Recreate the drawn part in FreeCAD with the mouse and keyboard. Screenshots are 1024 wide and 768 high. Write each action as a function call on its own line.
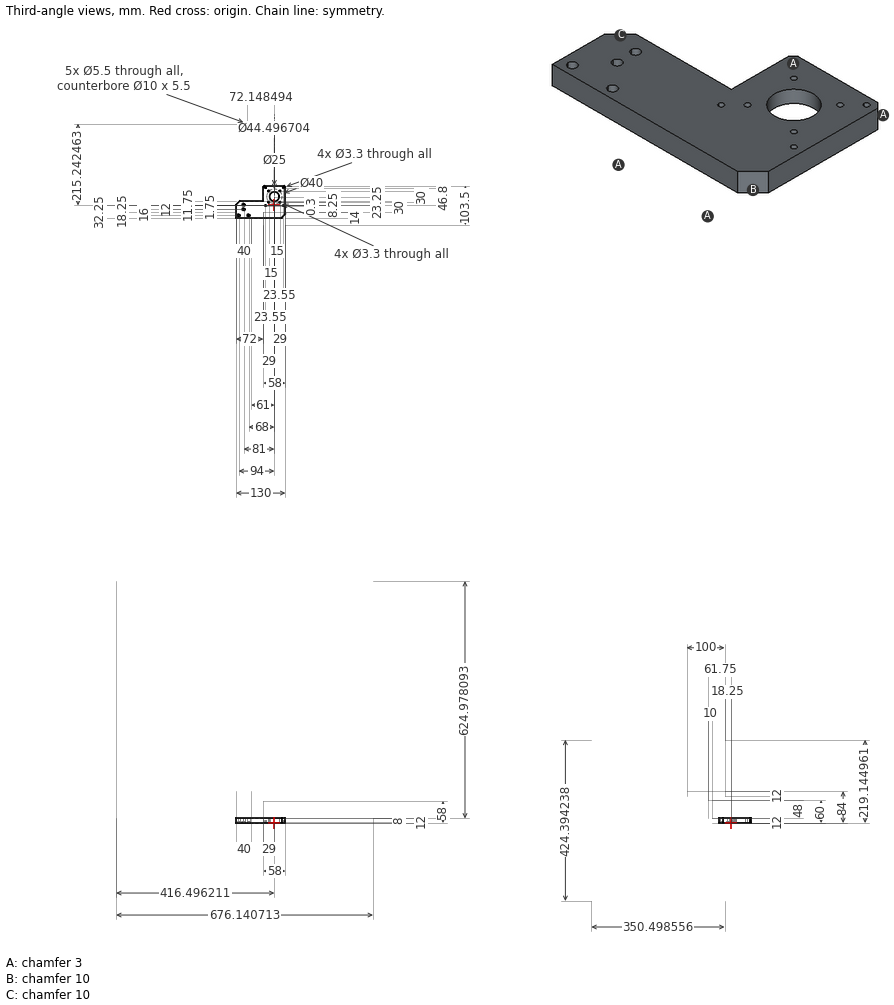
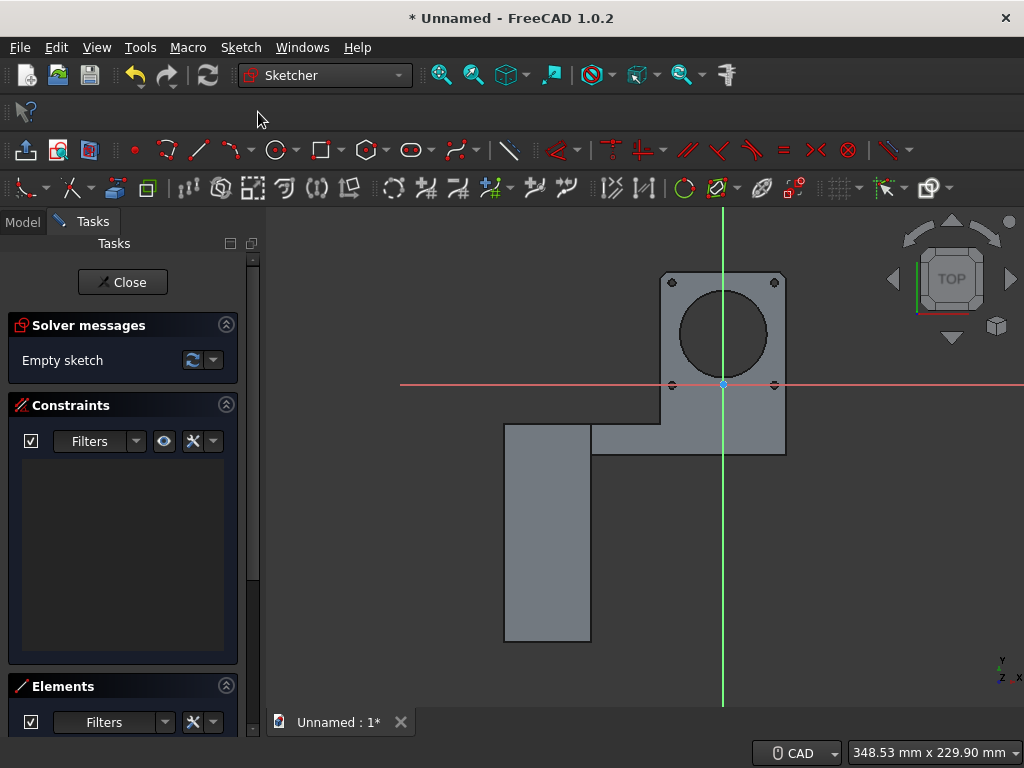
click(90, 150)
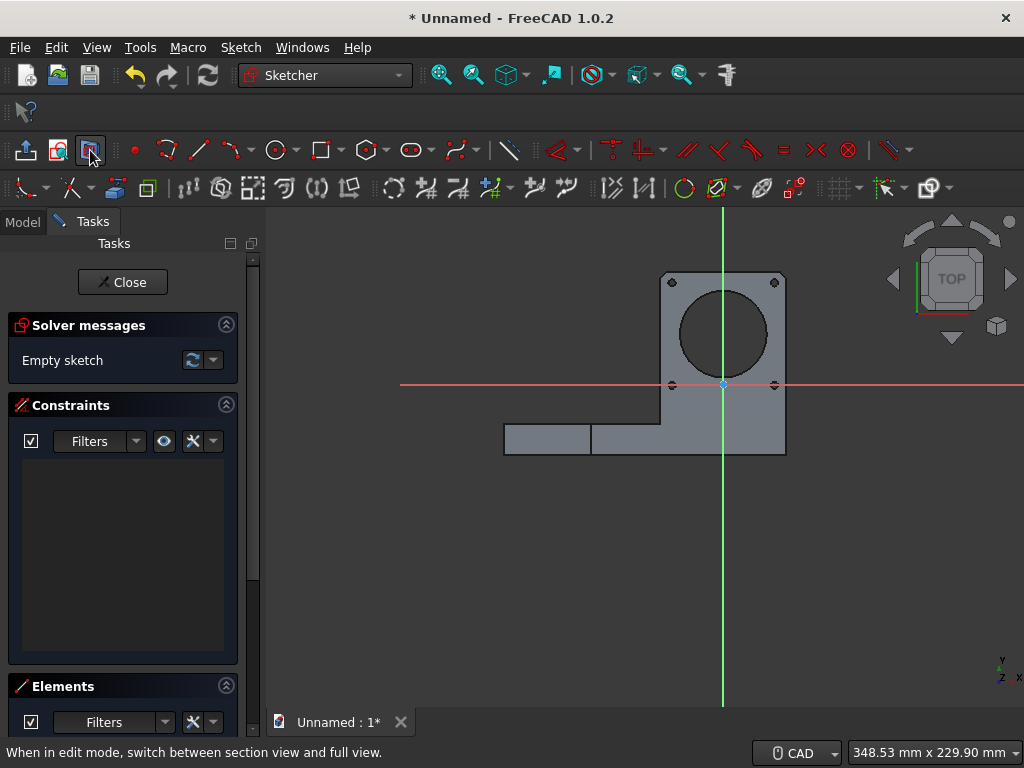
scroll(658, 312, up, 3)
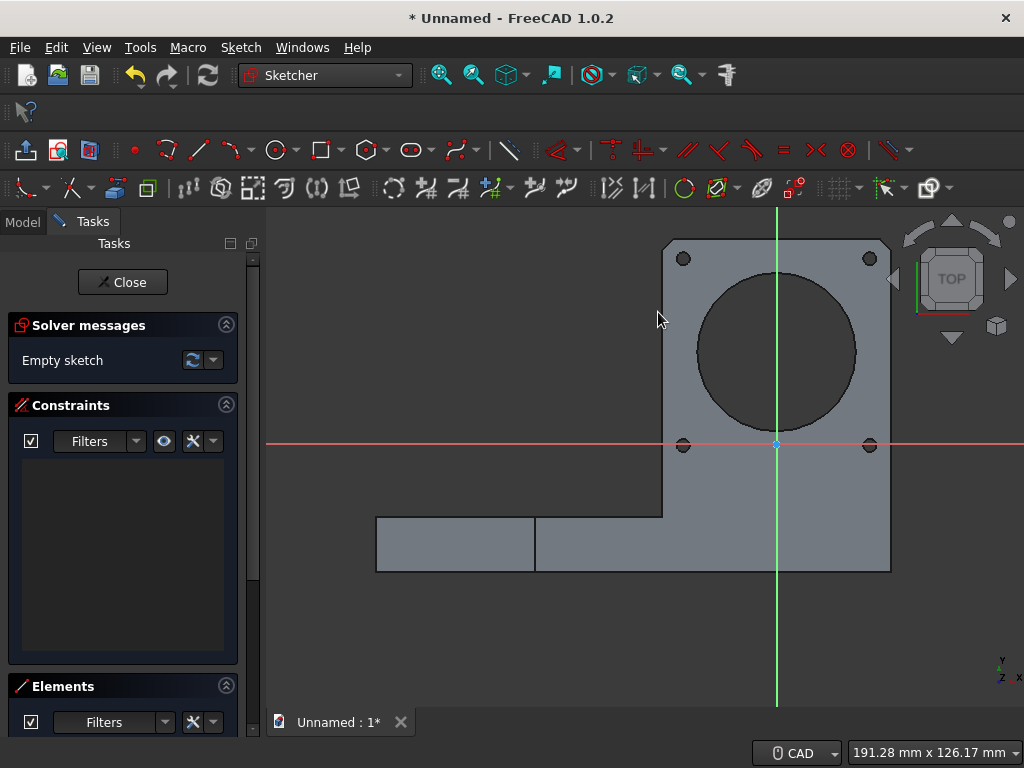
key(g)
key(r)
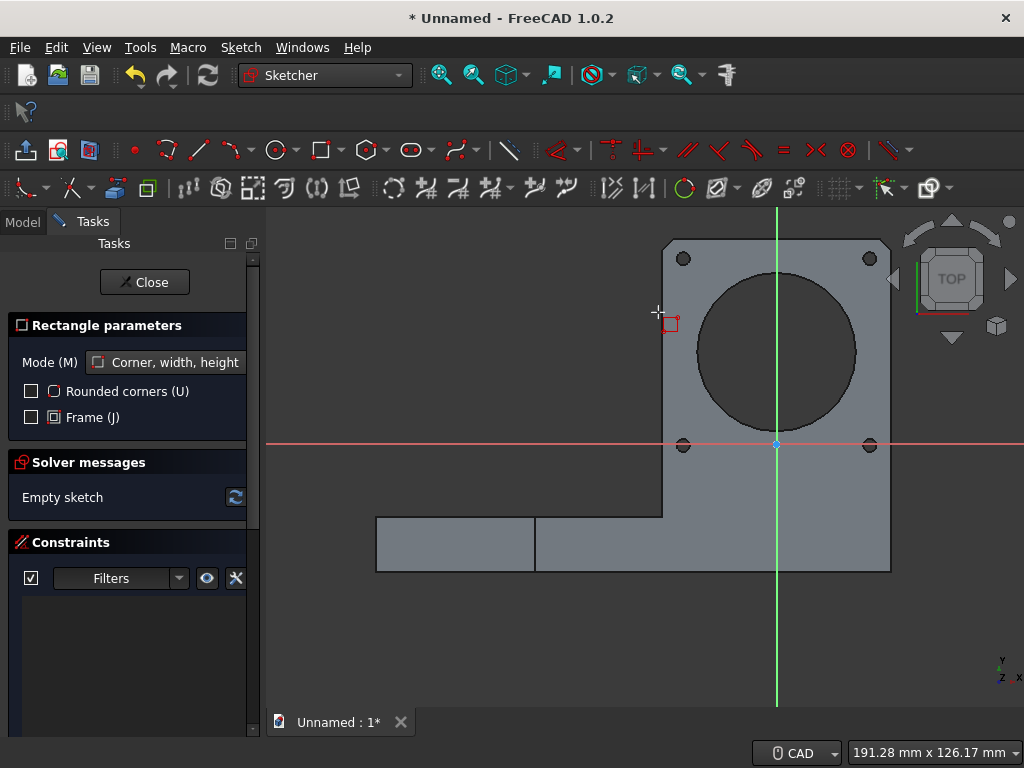
click(376, 398)
move(662, 517)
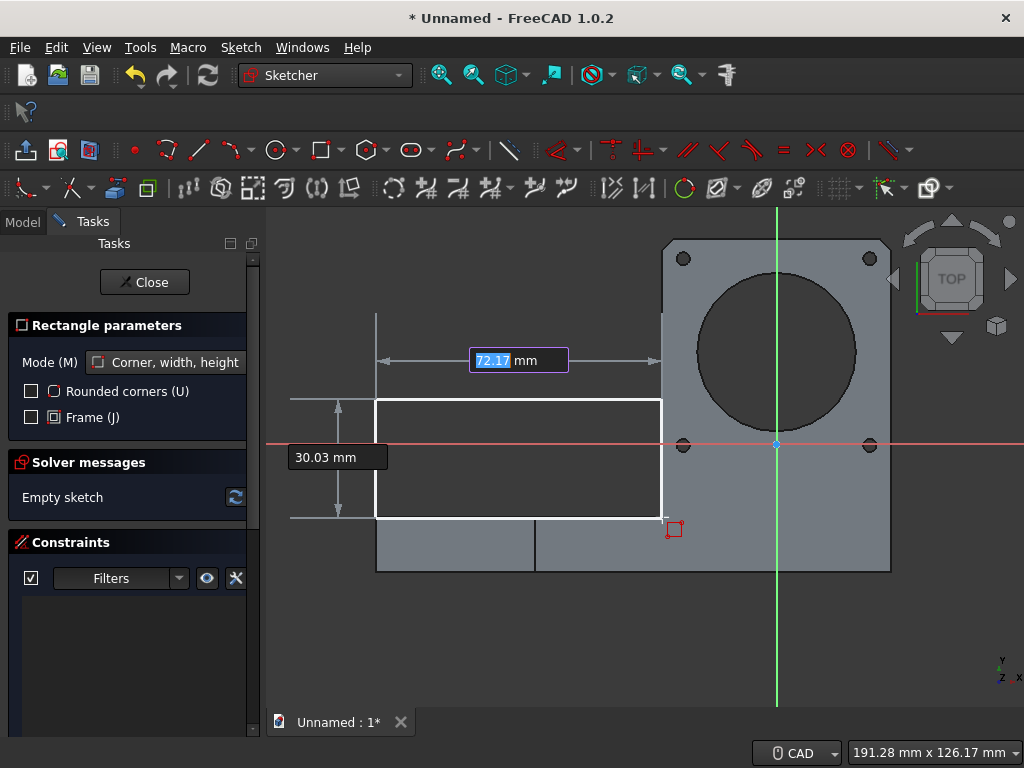
text(72)
key(Tab)
text(30)
key(Return)
key(Escape)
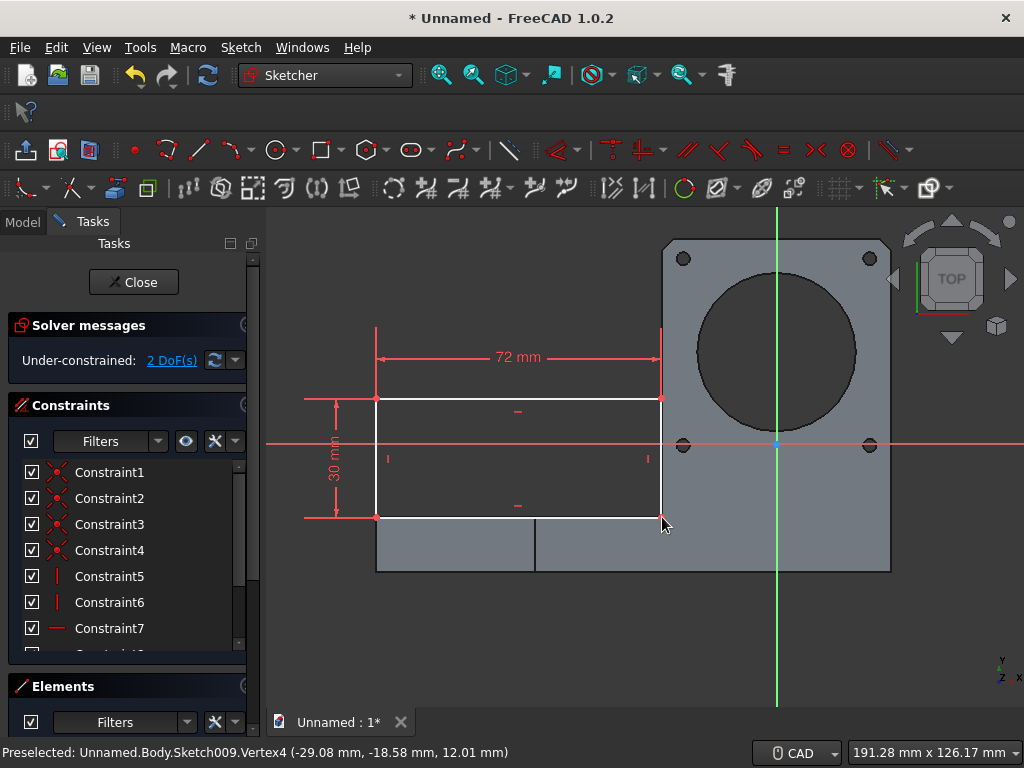
click(556, 150)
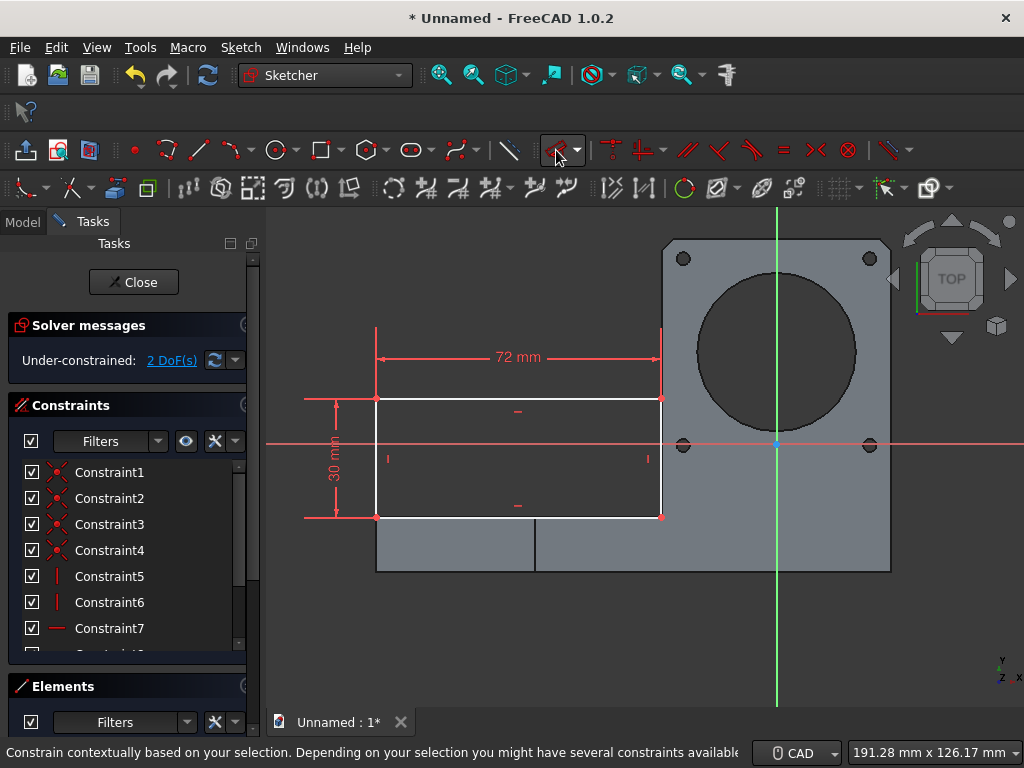
click(661, 518)
click(719, 552)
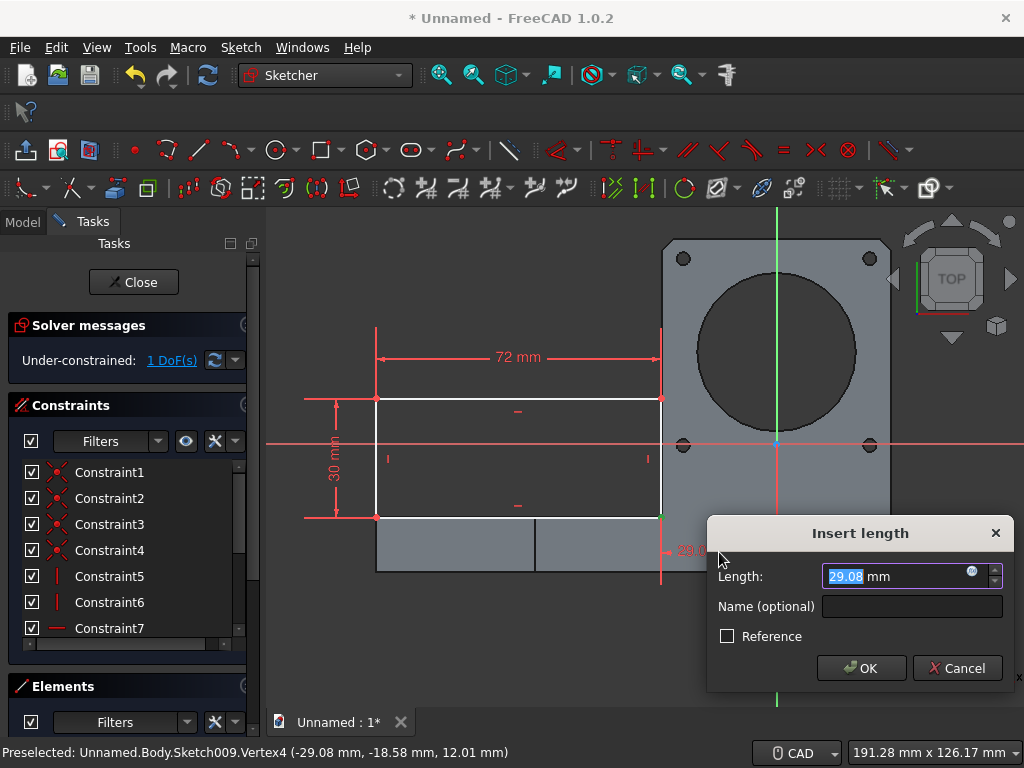
text(29)
key(Return)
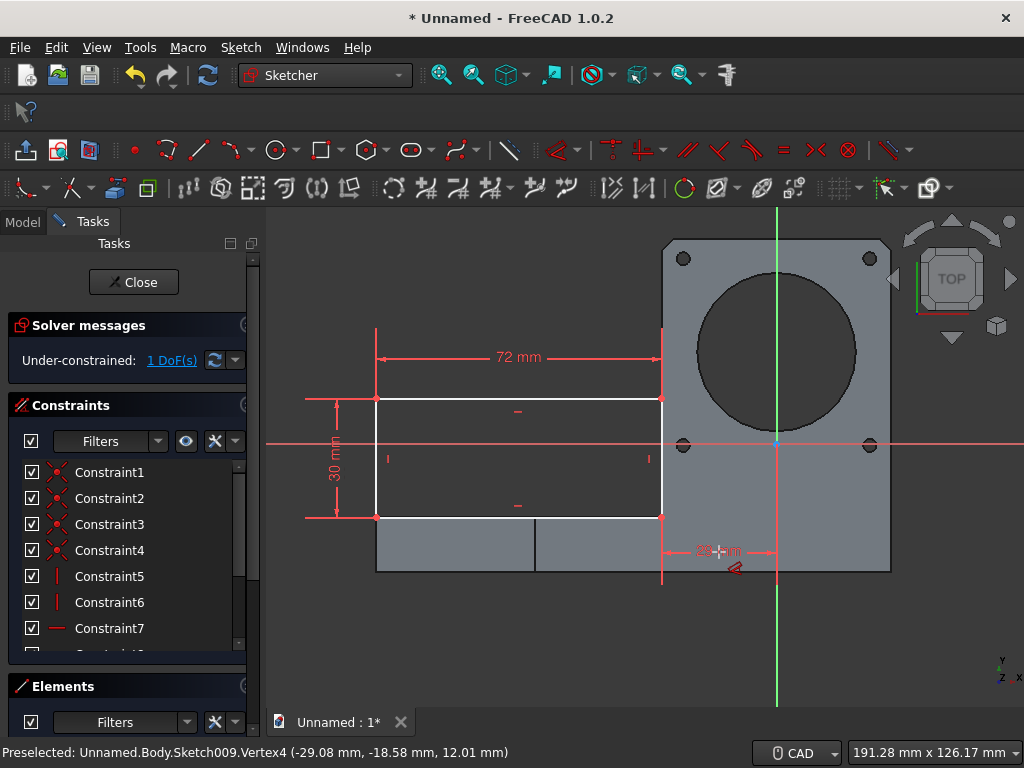
click(376, 399)
click(811, 422)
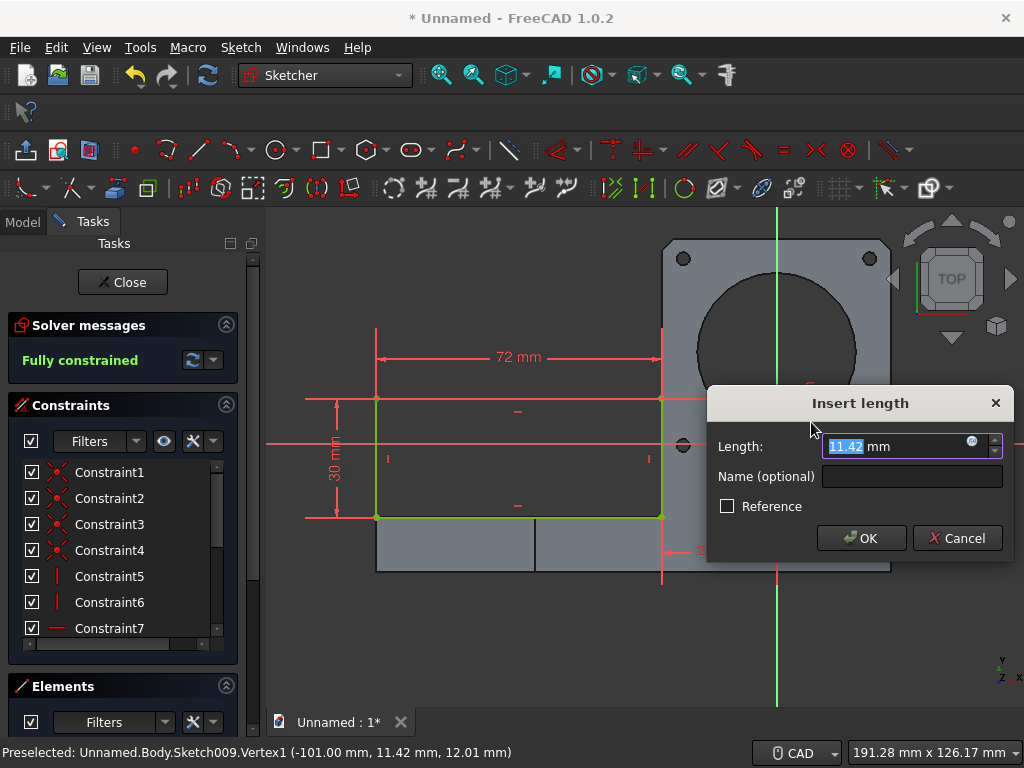
text(11.75)
key(Return)
key(Escape)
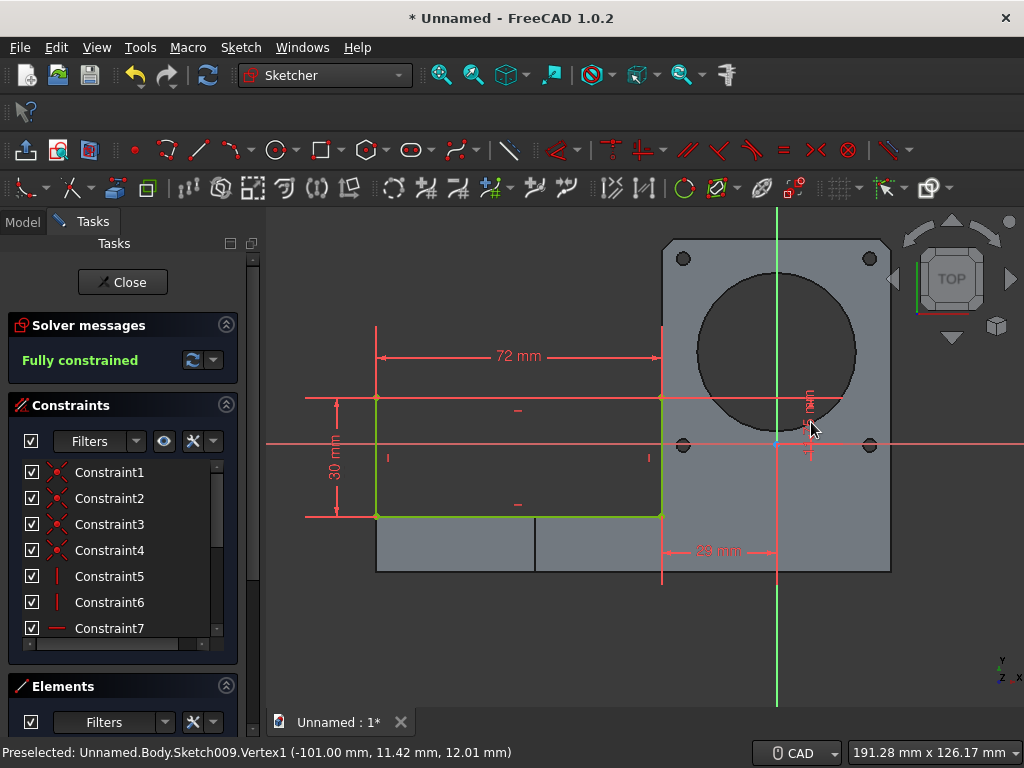
click(123, 282)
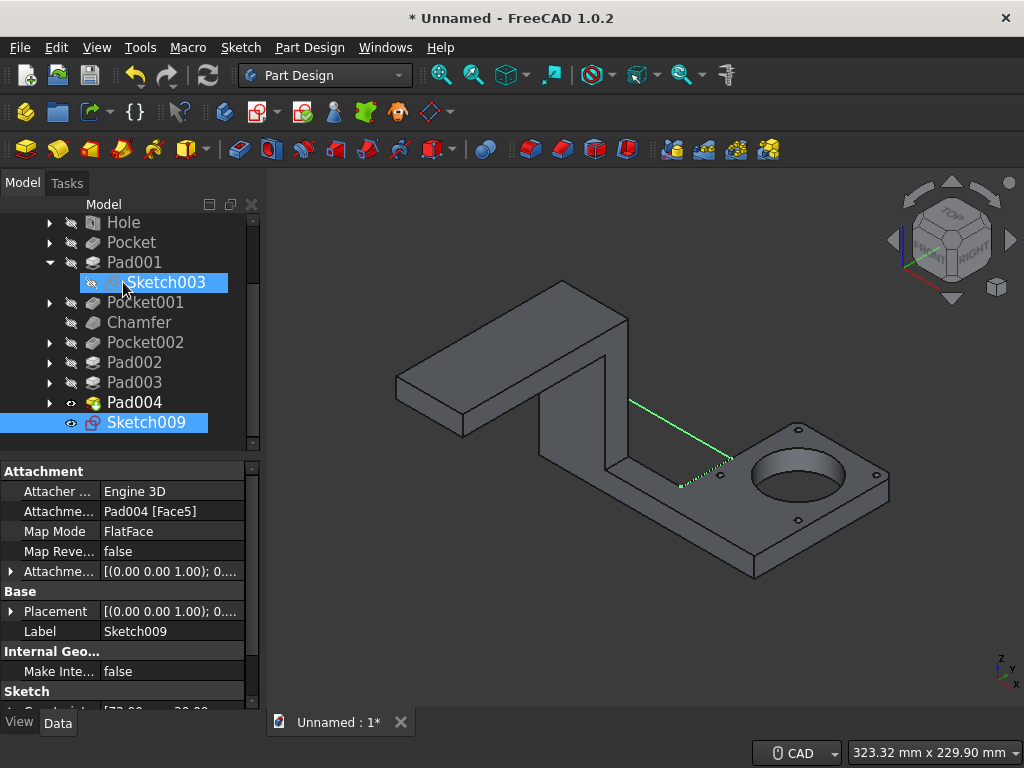
click(26, 150)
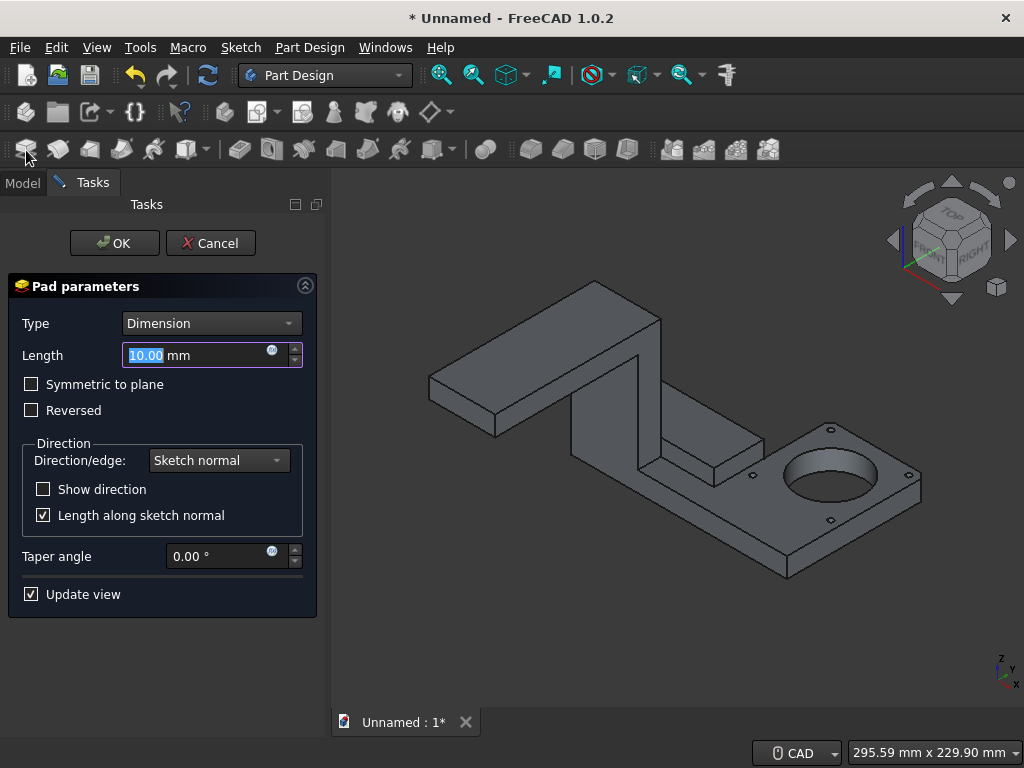
text(12)
key(Tab)